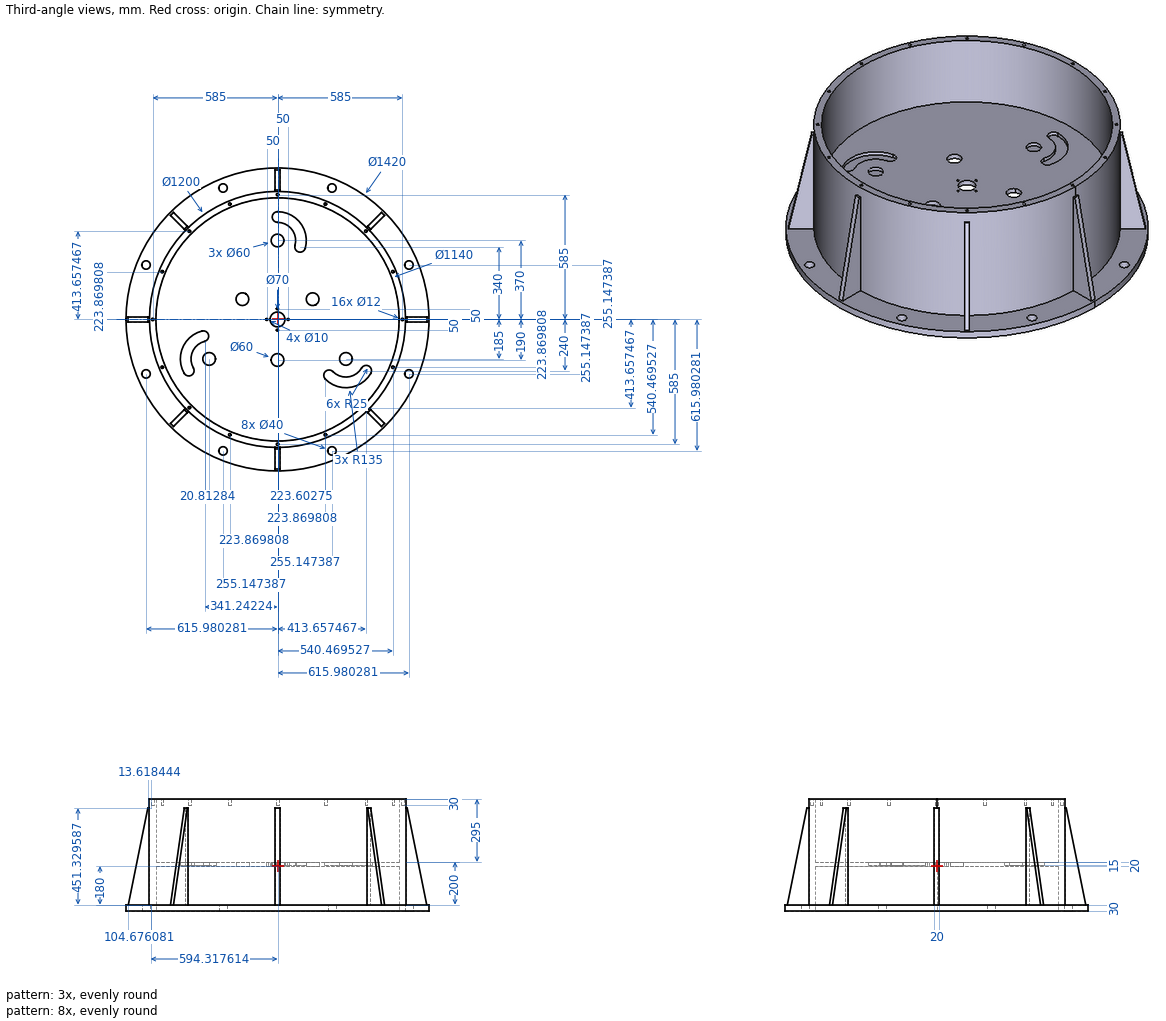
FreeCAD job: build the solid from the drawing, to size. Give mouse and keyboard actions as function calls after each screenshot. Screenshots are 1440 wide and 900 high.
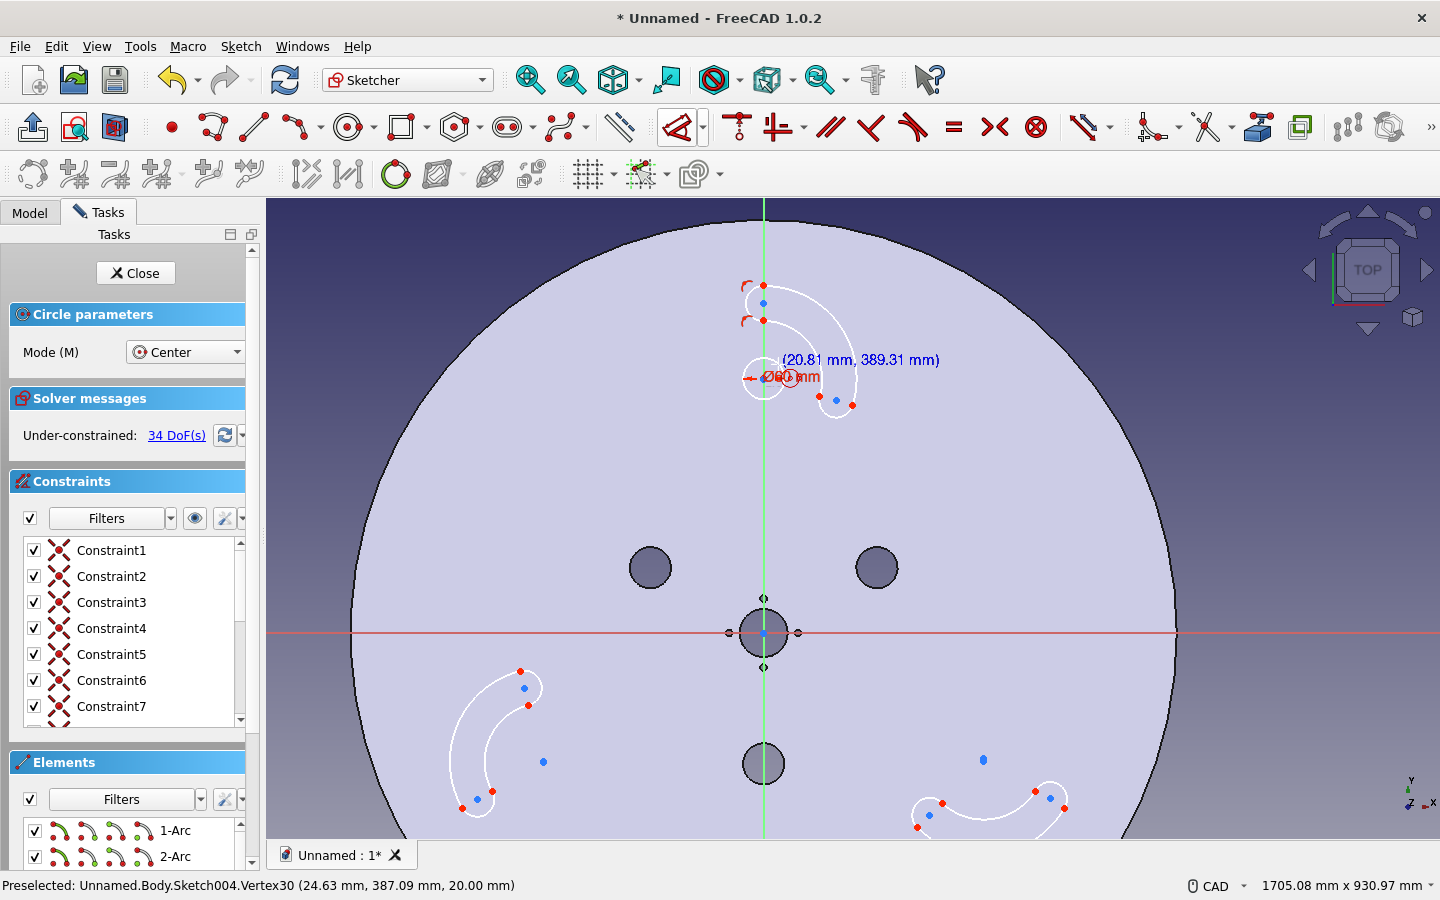
click(984, 760)
move(999, 746)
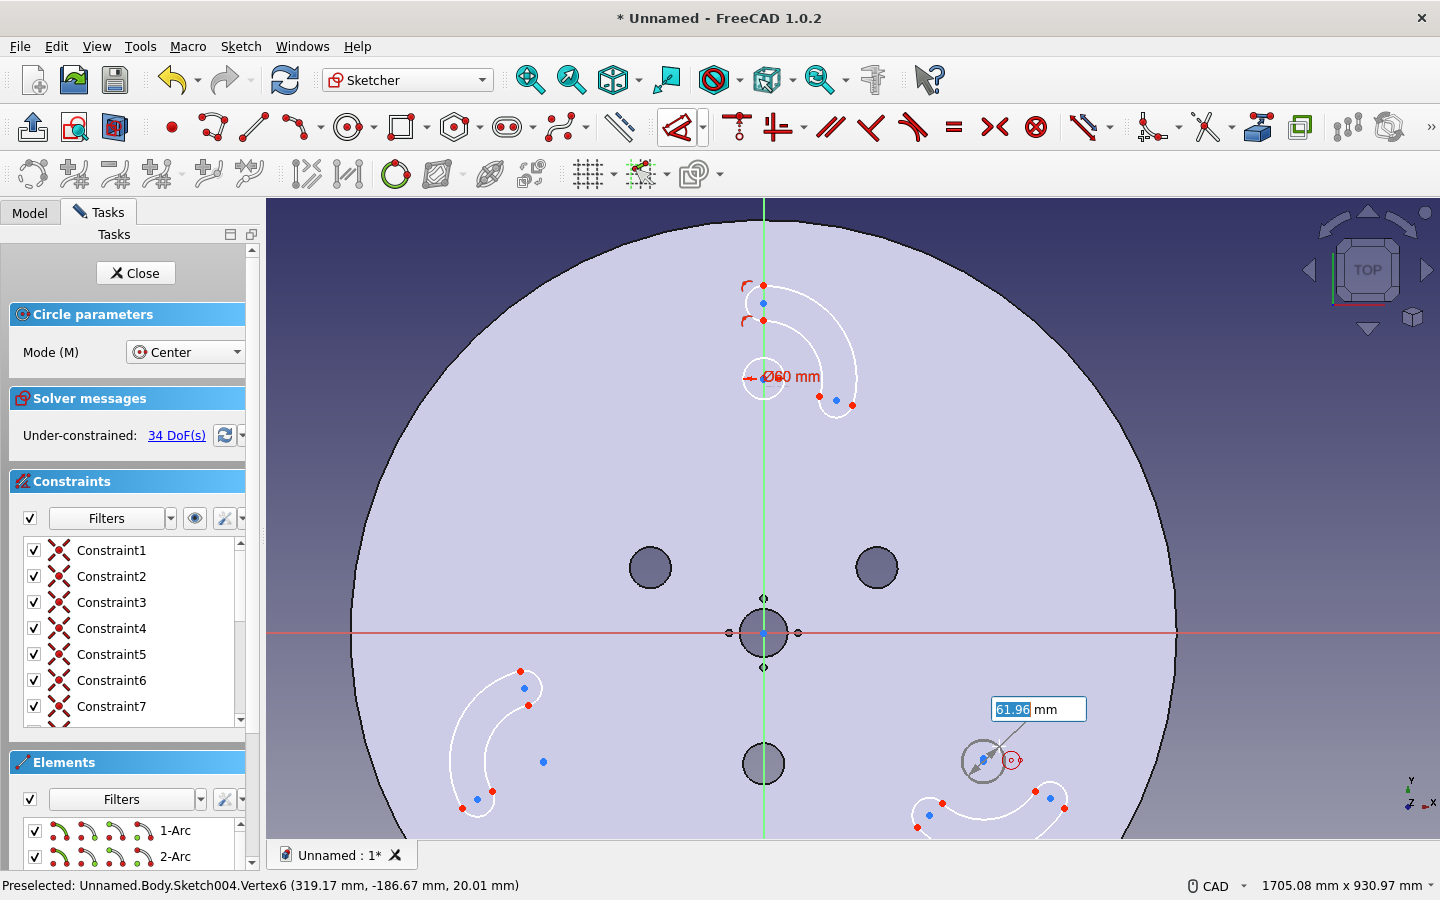
text(60)
key(Return)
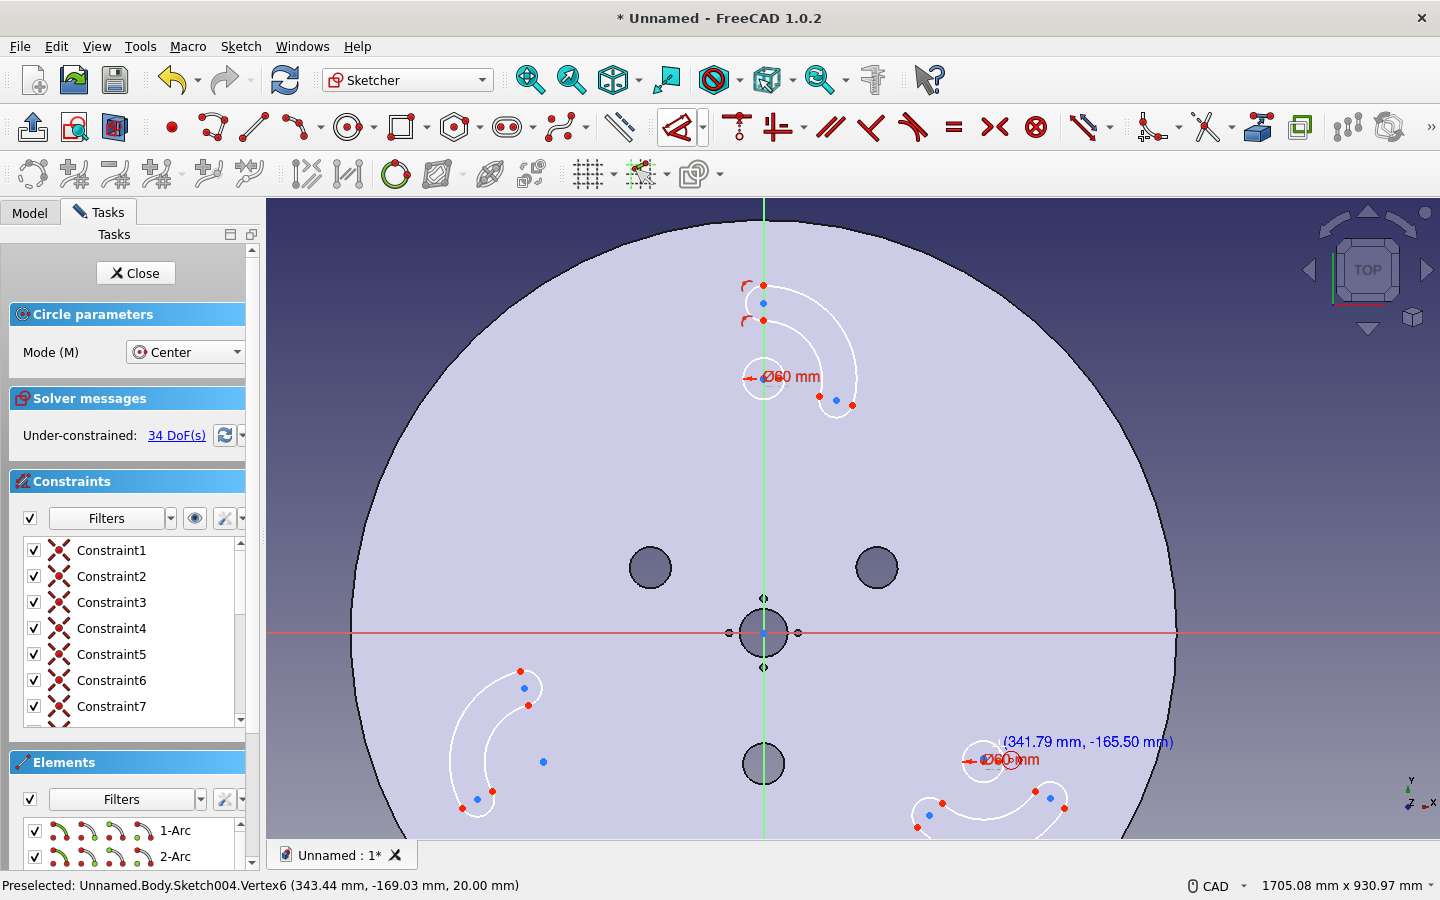
click(543, 760)
move(558, 746)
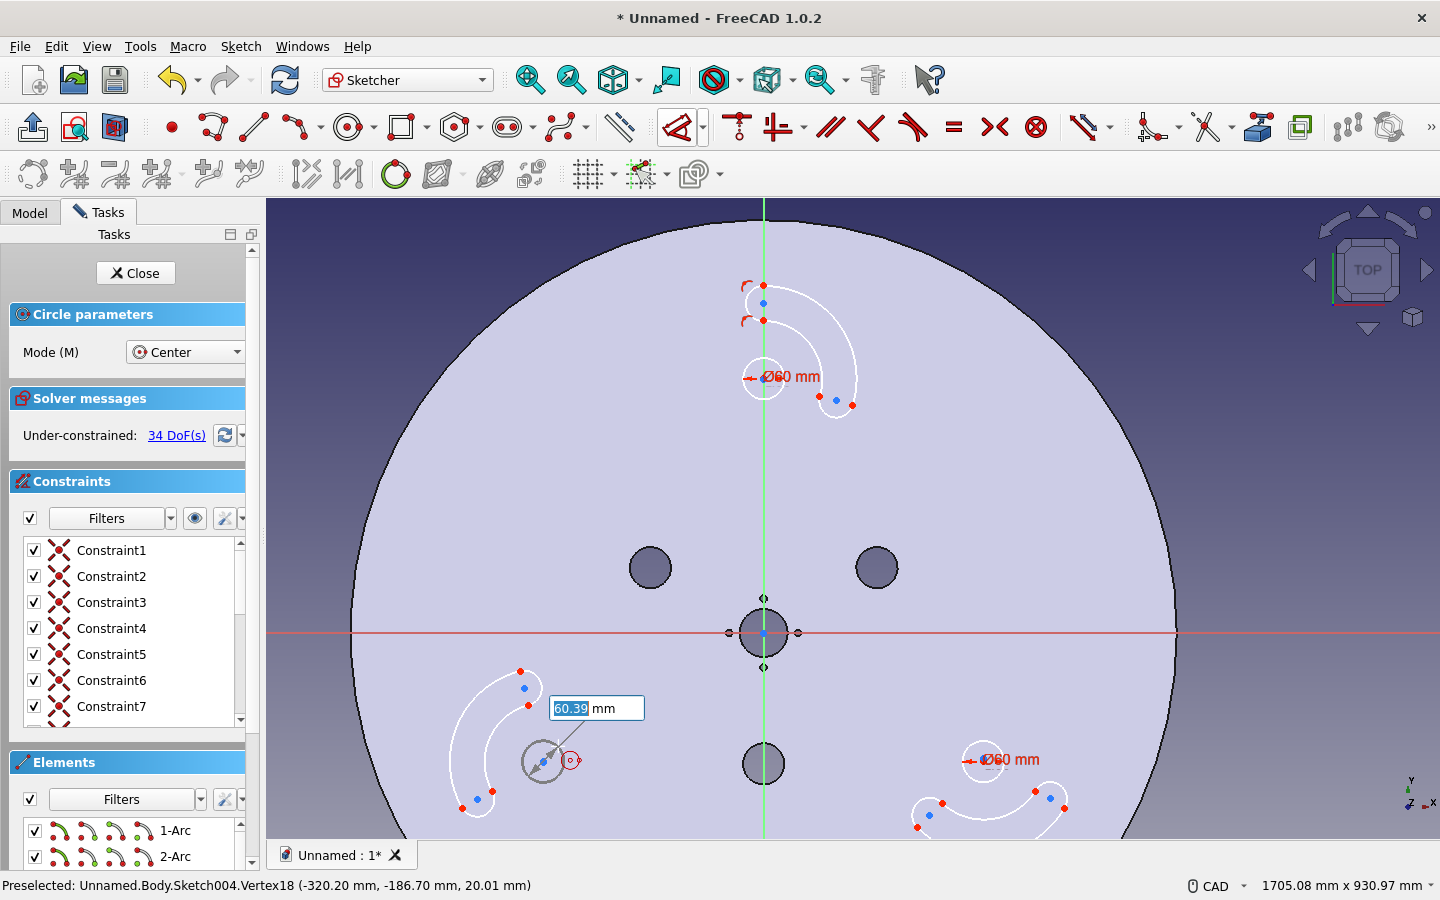
text(60)
key(Return)
key(Escape)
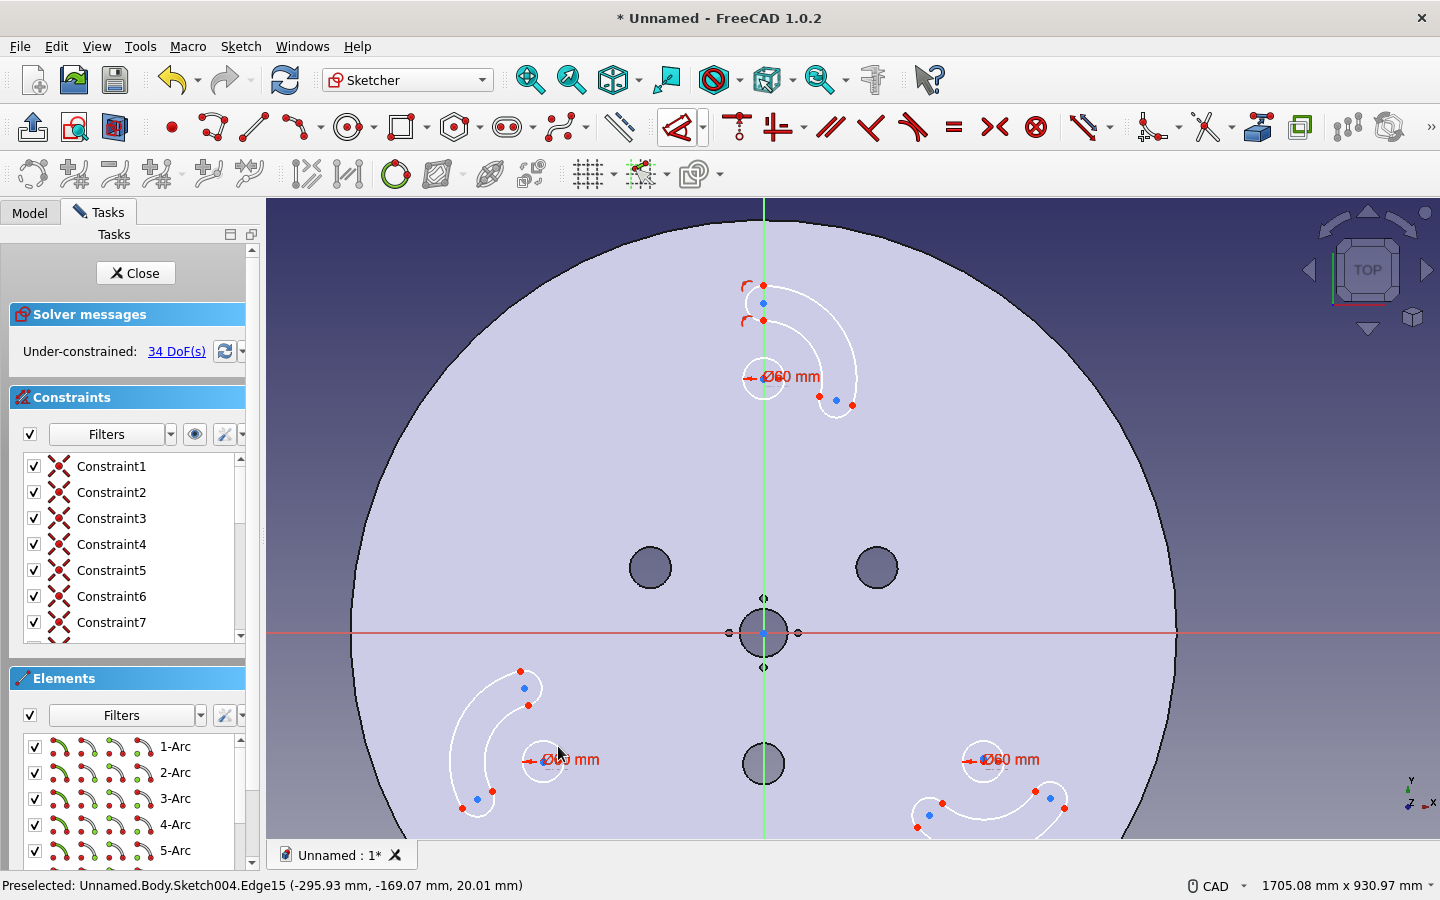
click(928, 798)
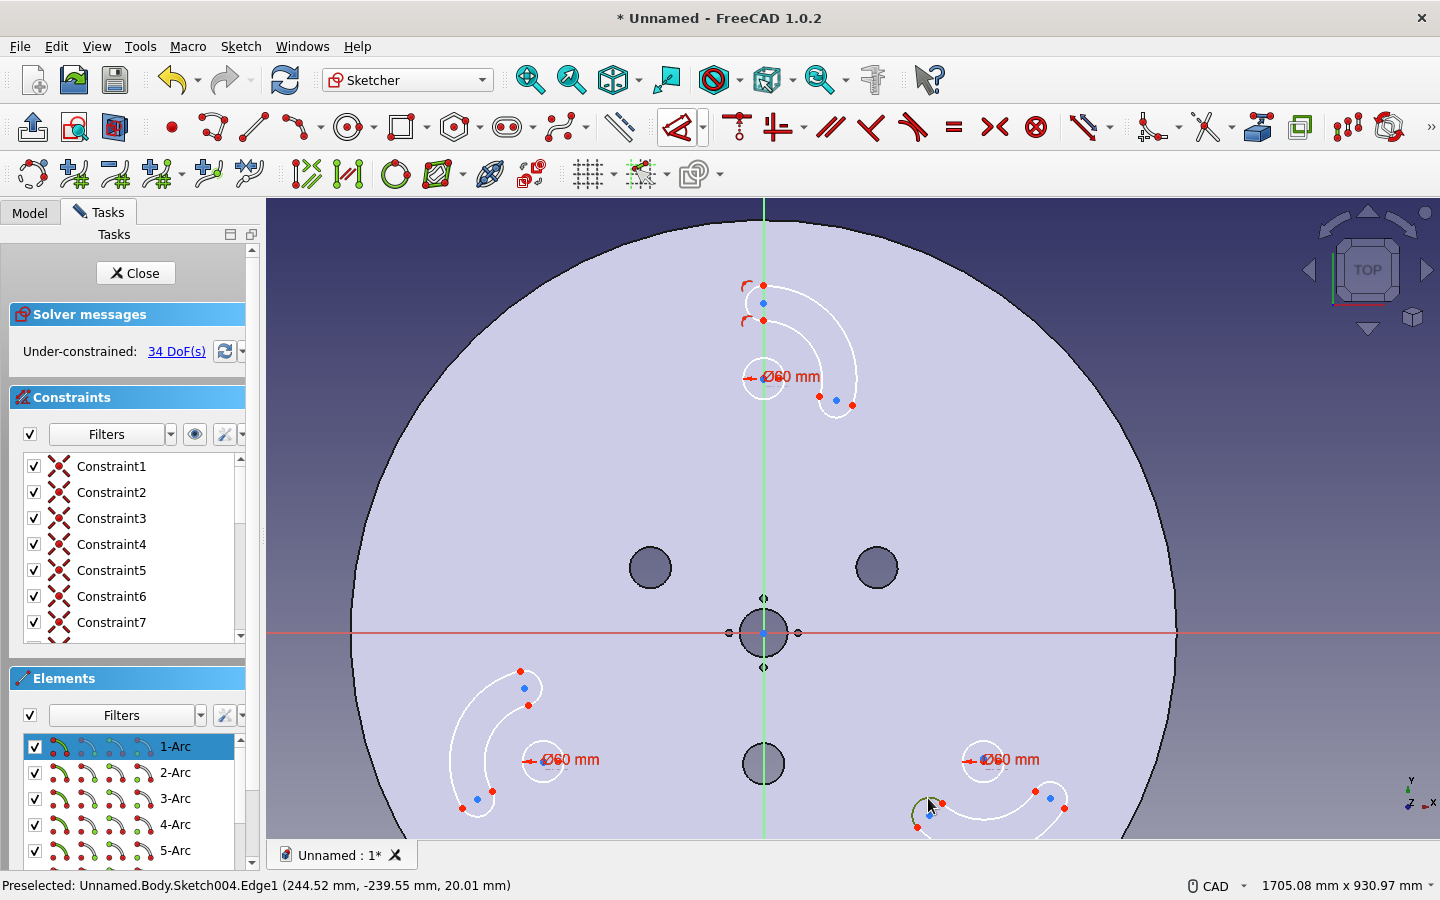
scroll(832, 416, down, 2)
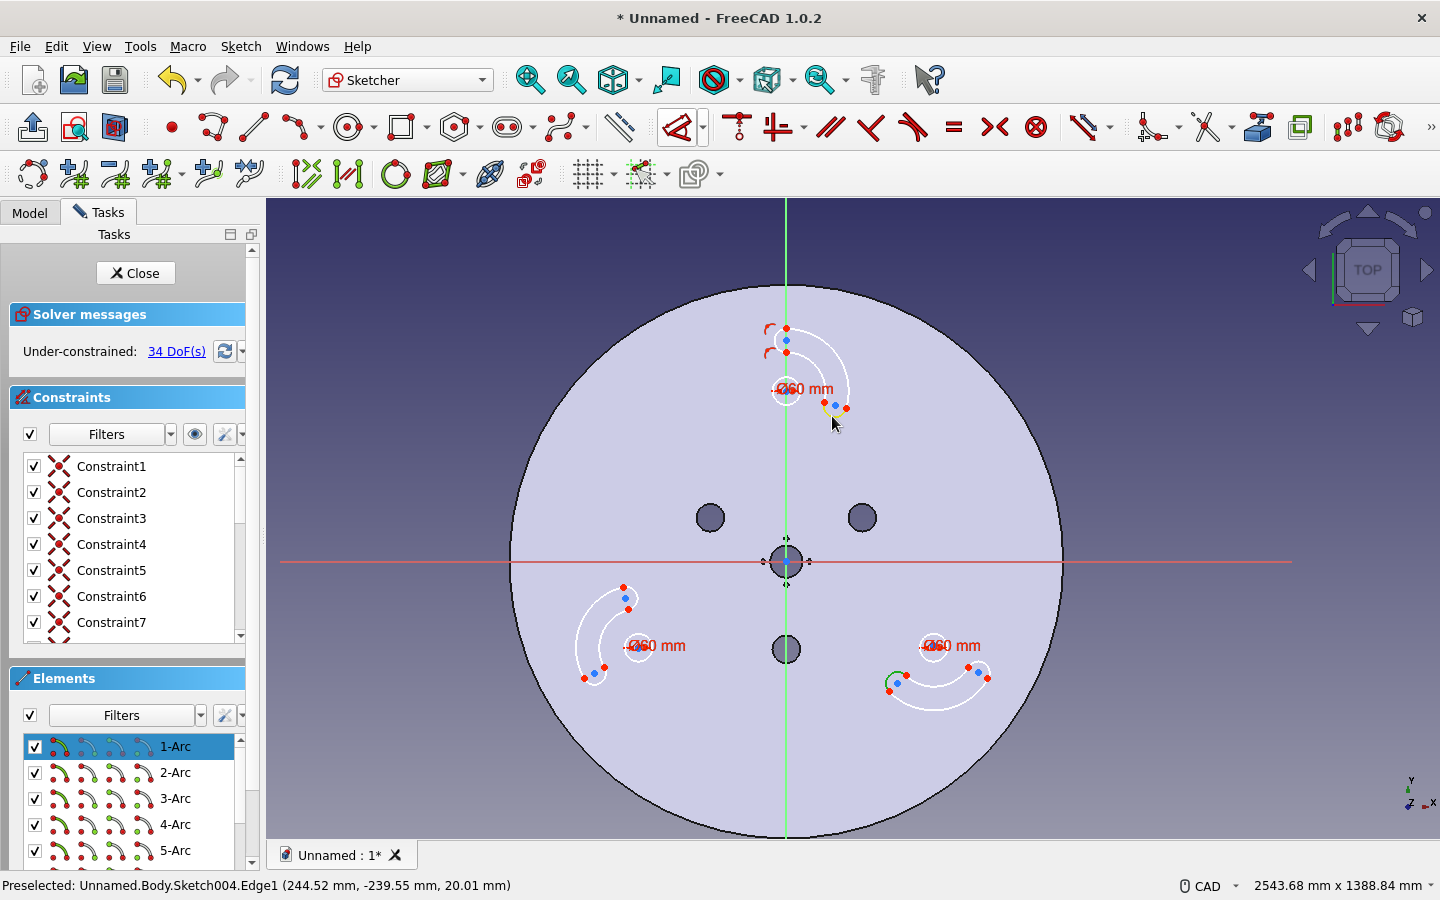
click(919, 709)